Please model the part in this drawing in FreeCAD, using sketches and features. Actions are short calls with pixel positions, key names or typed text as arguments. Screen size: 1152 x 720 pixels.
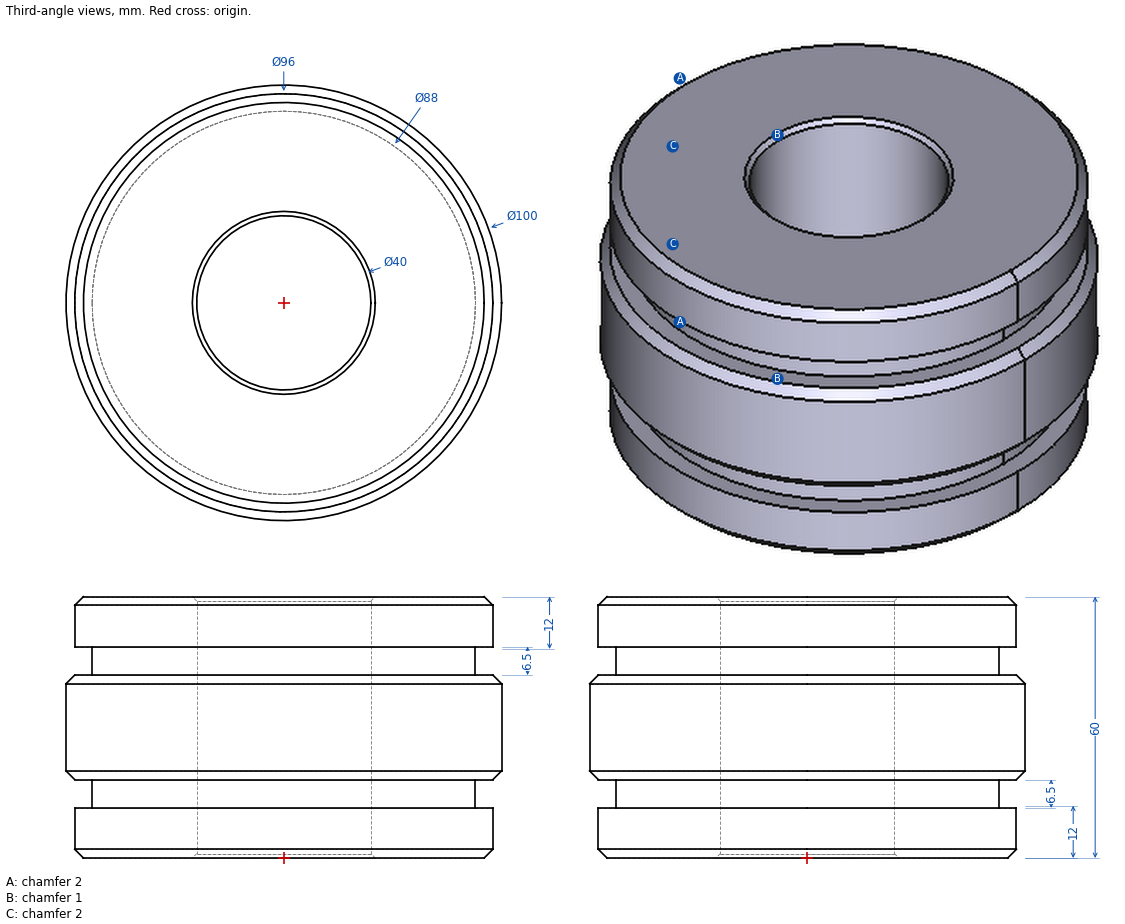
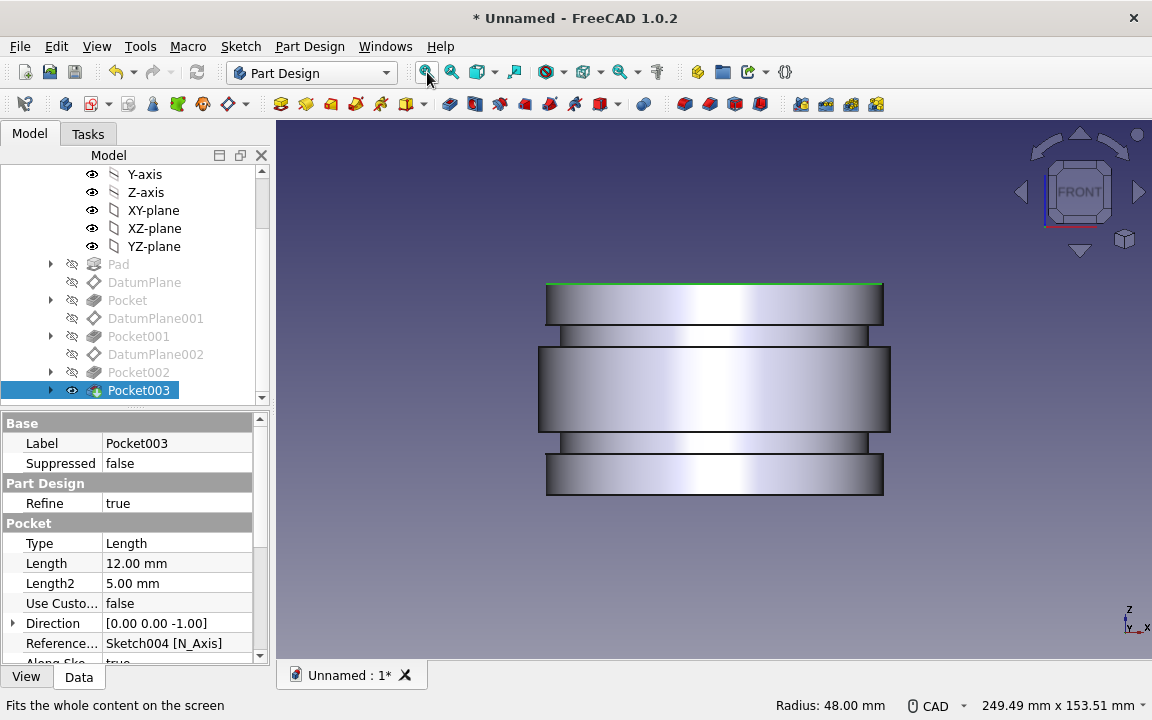
click(578, 494, ctrl)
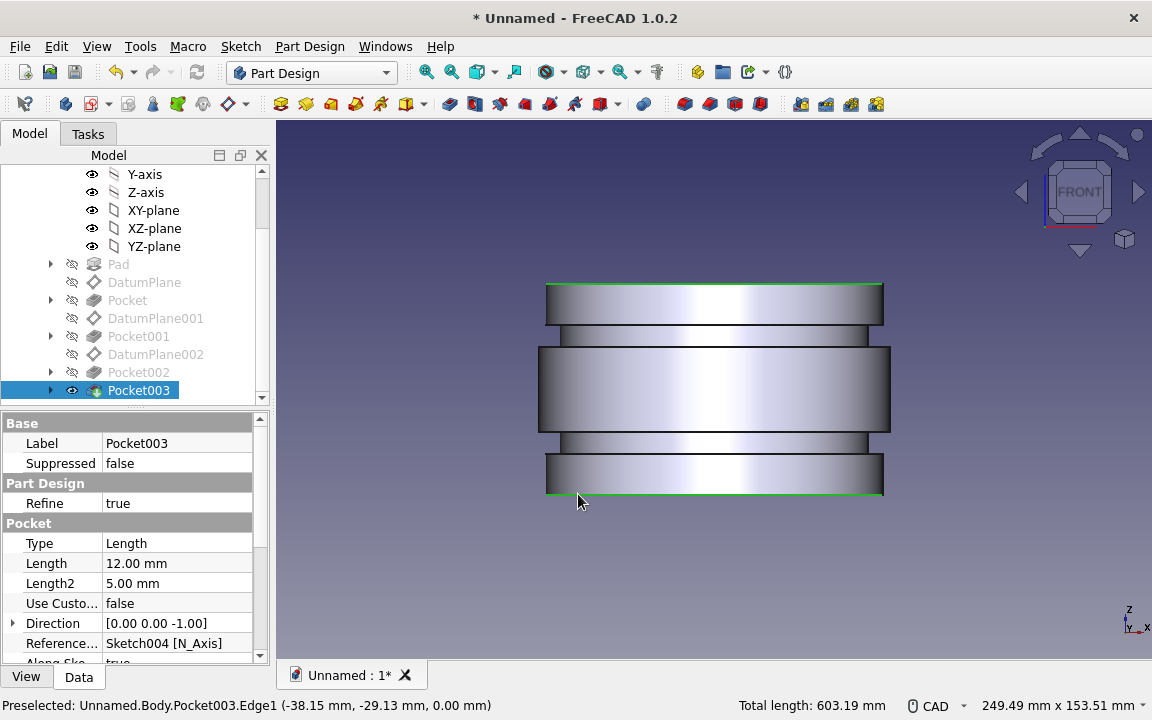
click(710, 104)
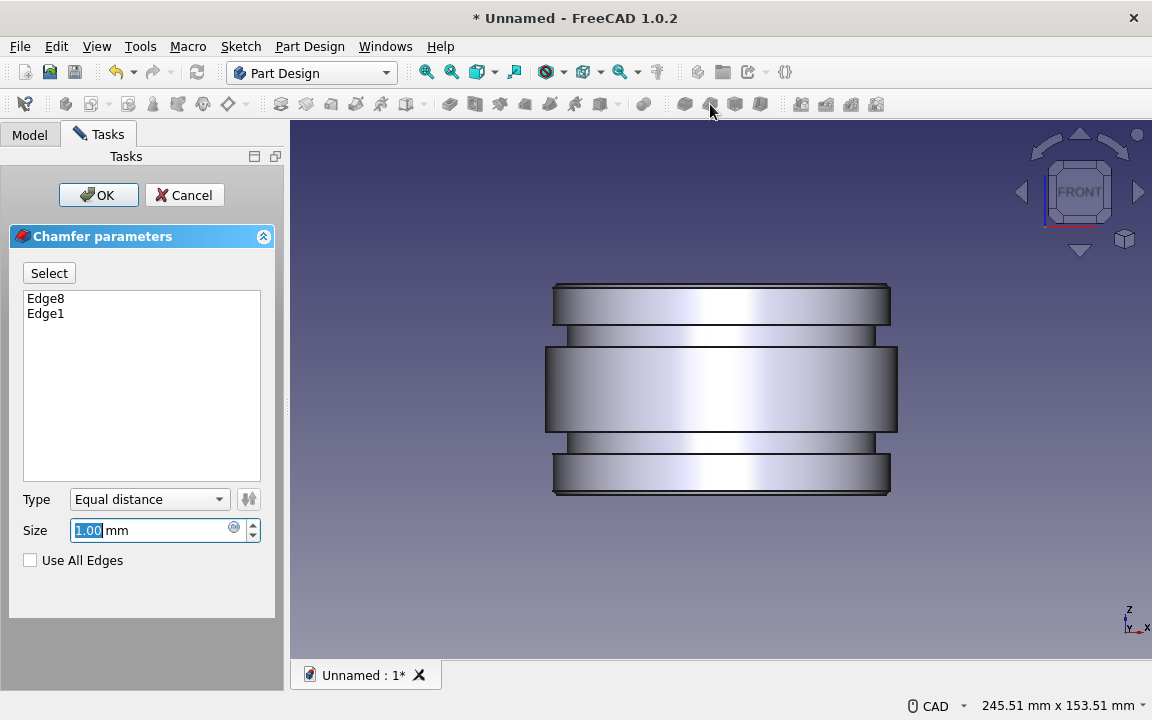
text(2)
key(Tab)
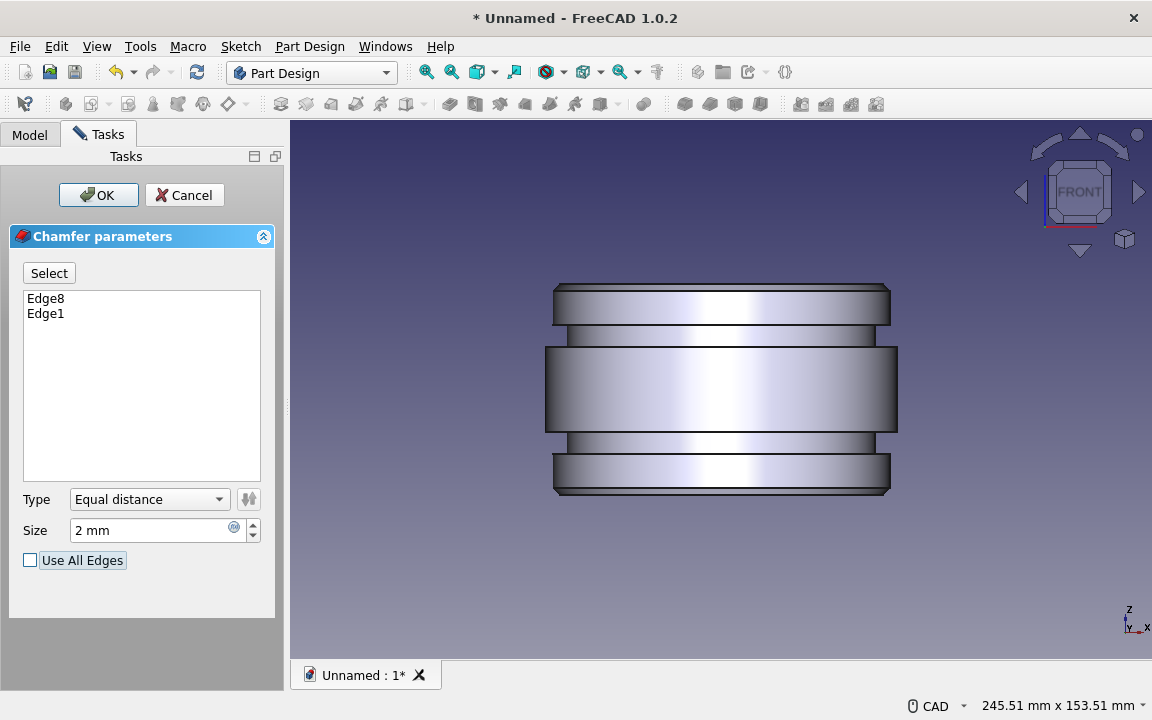
click(99, 195)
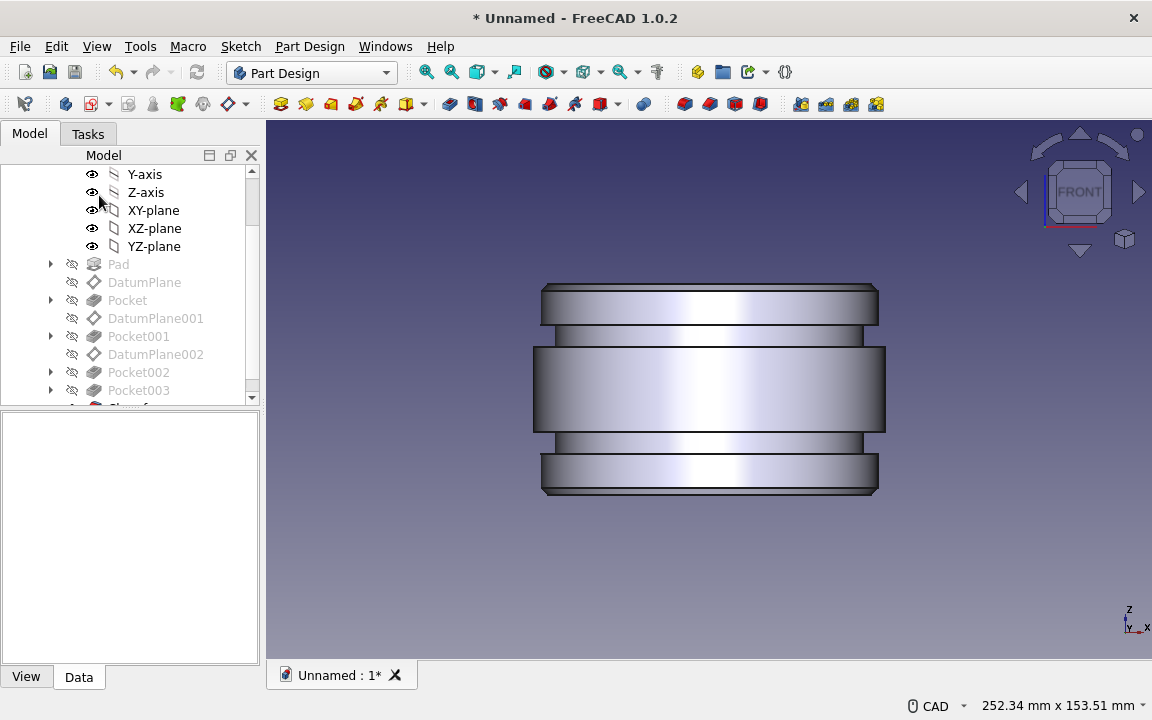
click(427, 72)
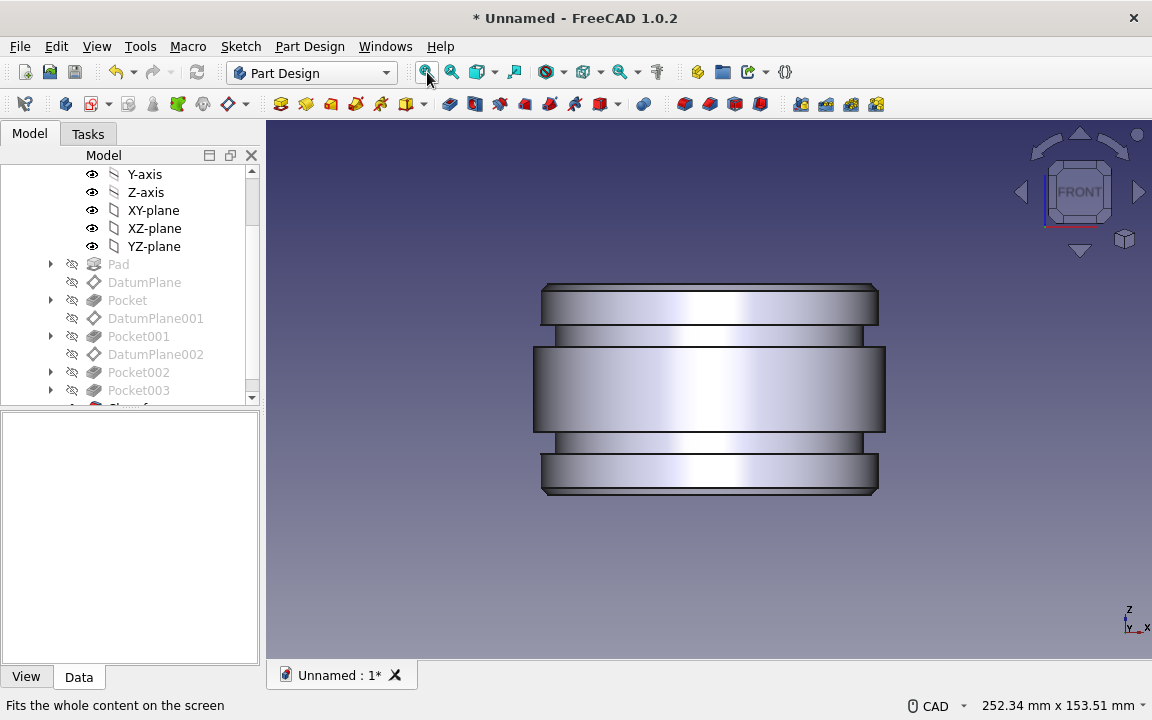
key(0)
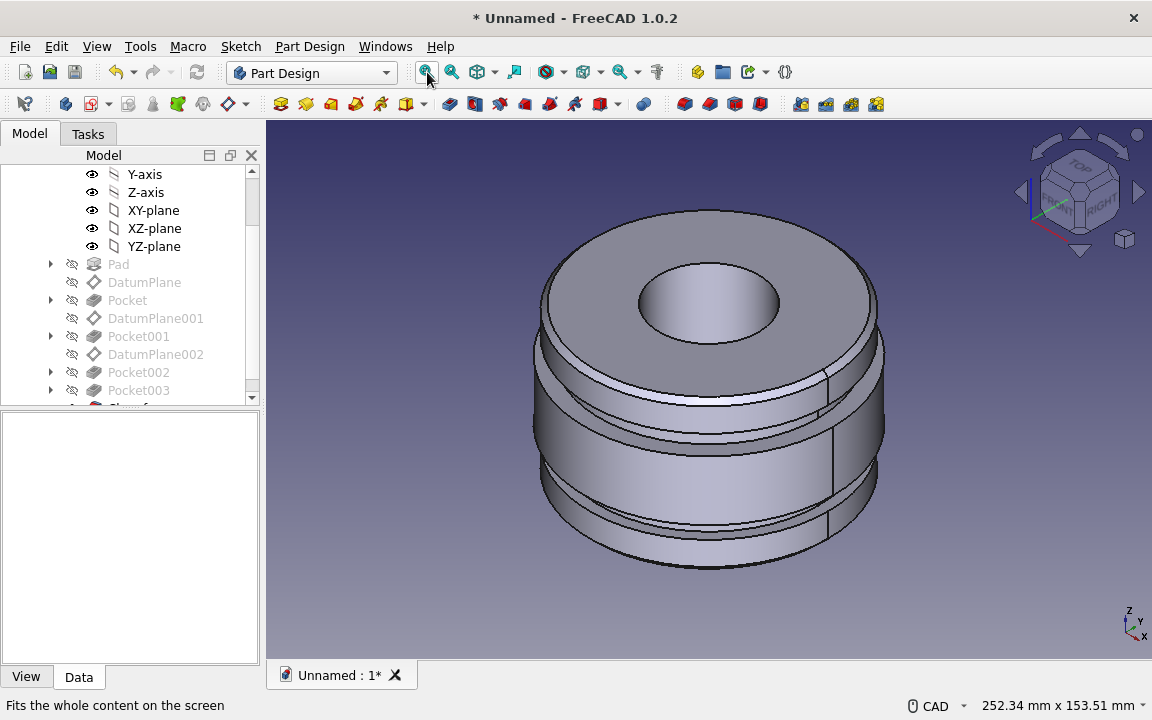
click(659, 274)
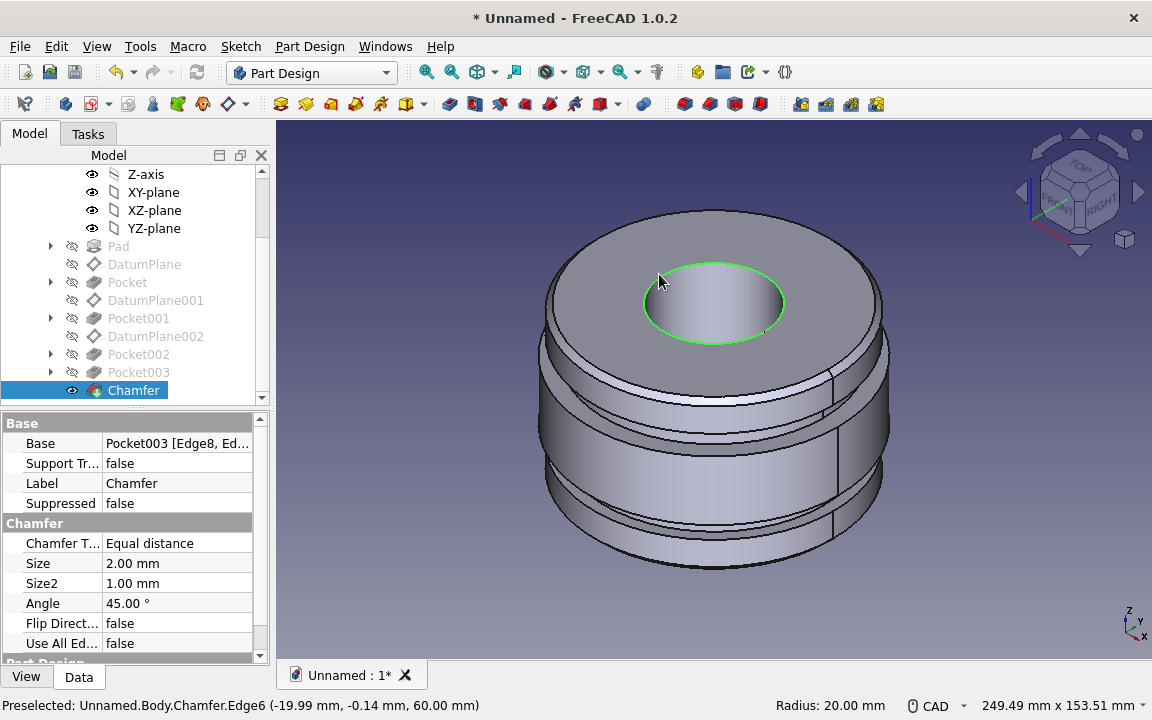
key(2)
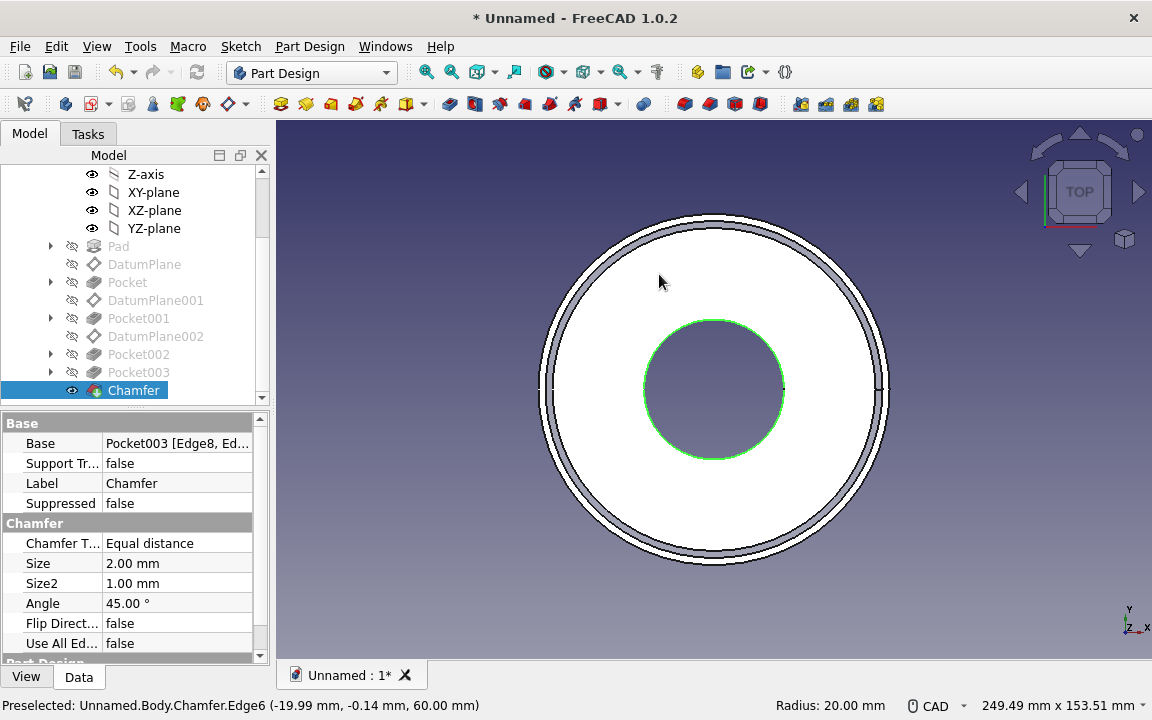
key(1)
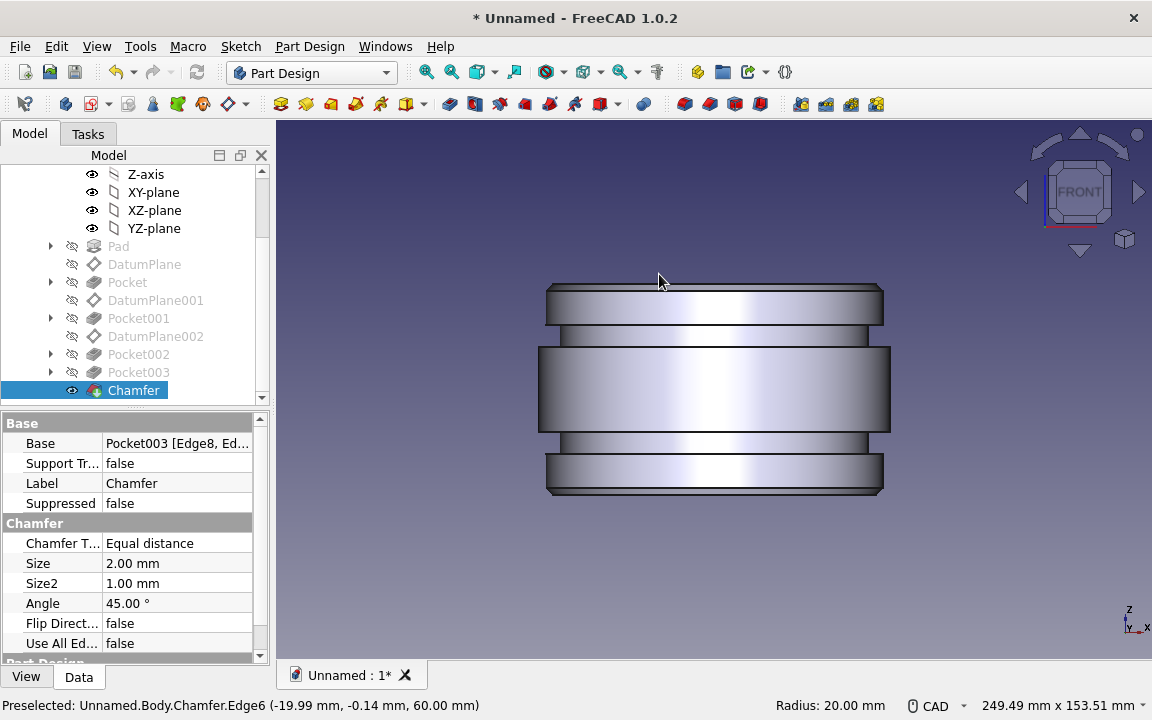
click(427, 72)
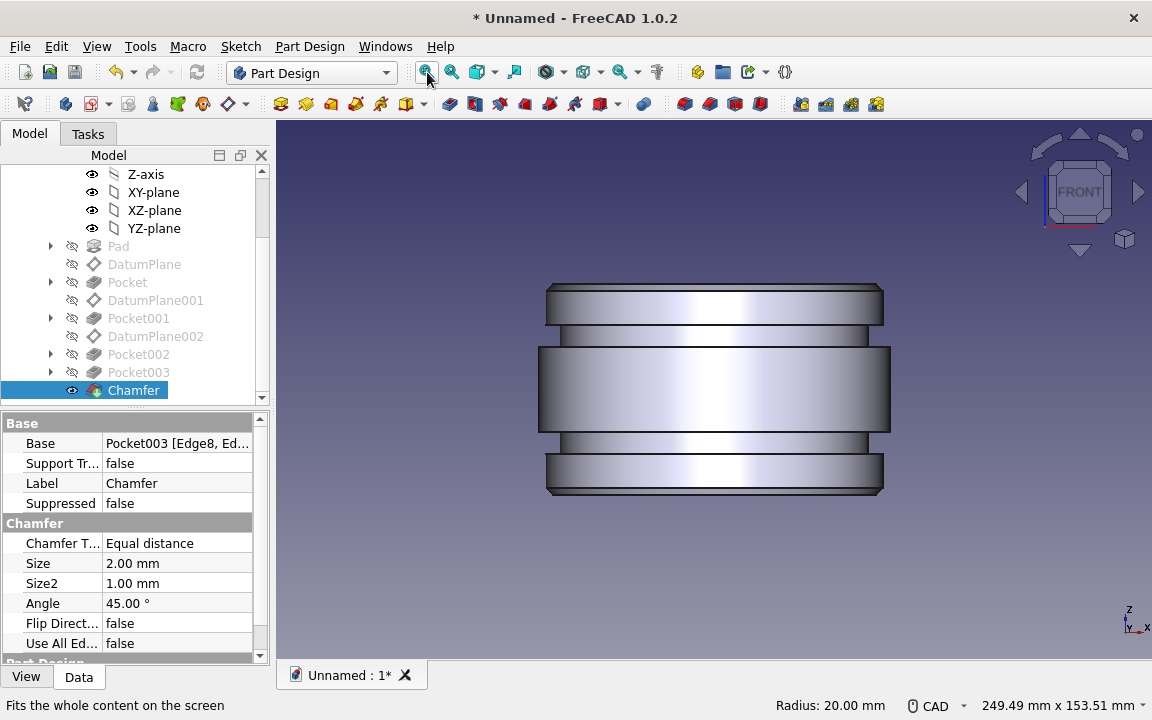
key(3)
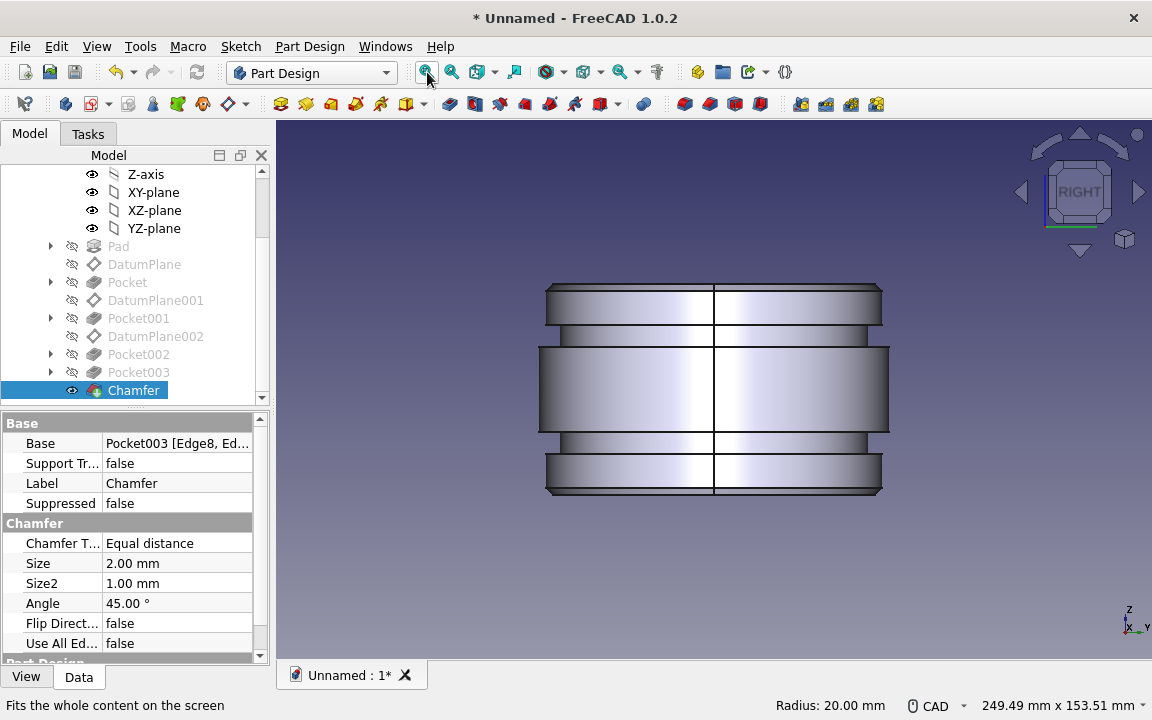
click(427, 72)